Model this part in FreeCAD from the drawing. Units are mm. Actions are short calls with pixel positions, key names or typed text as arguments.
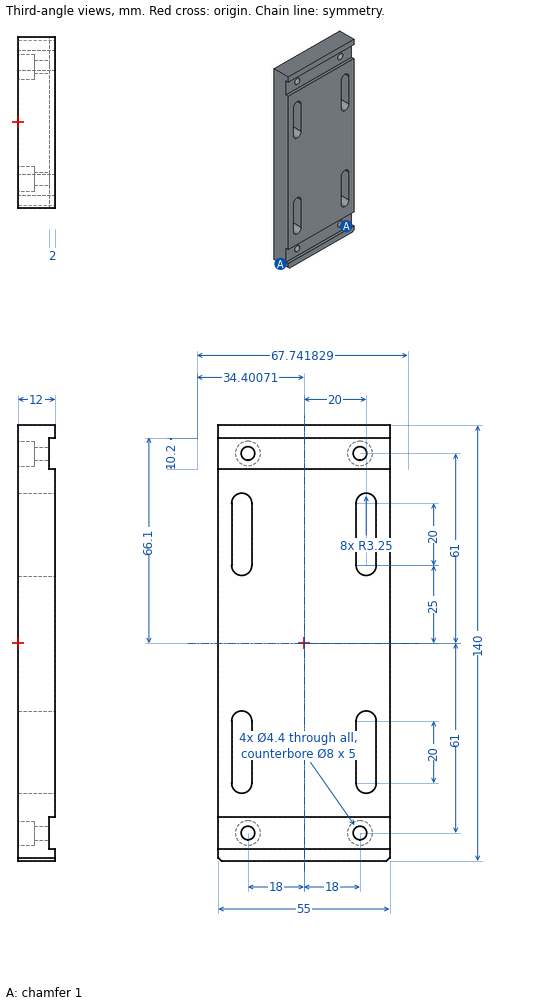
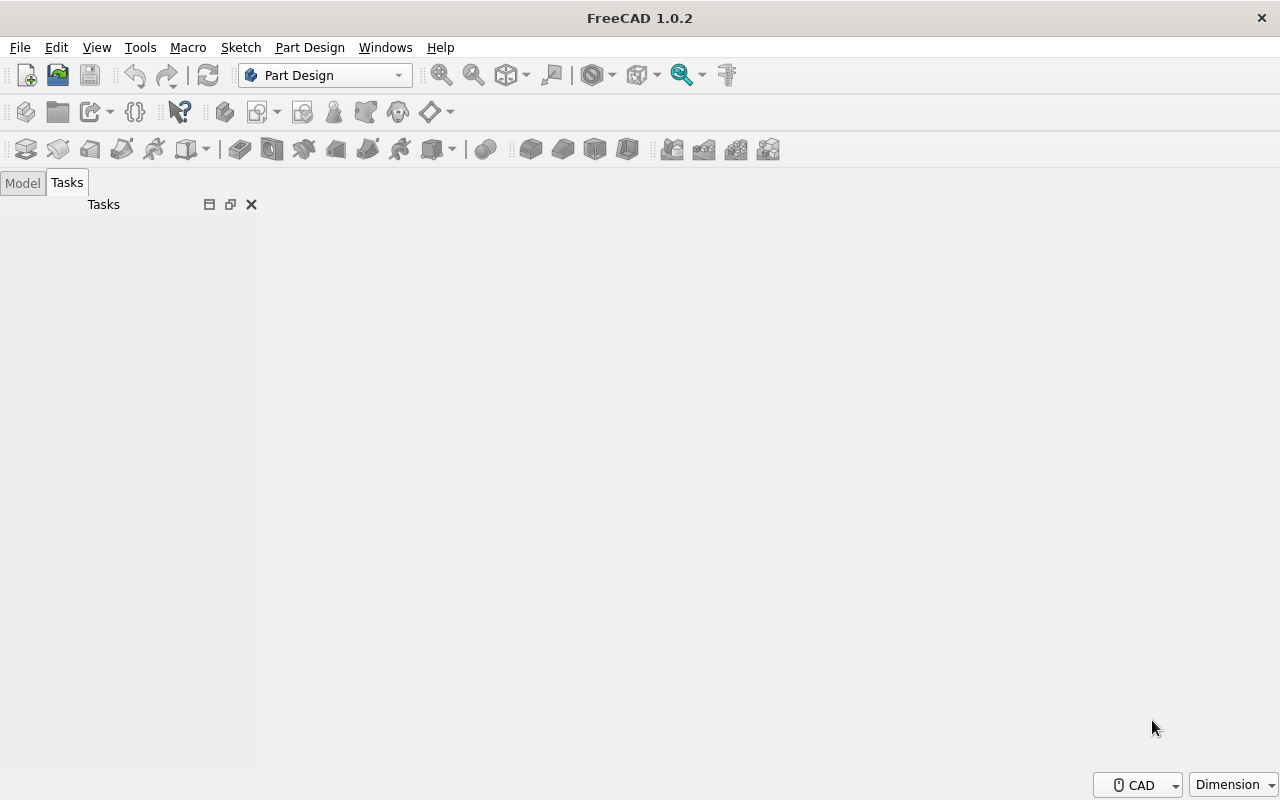
click(26, 76)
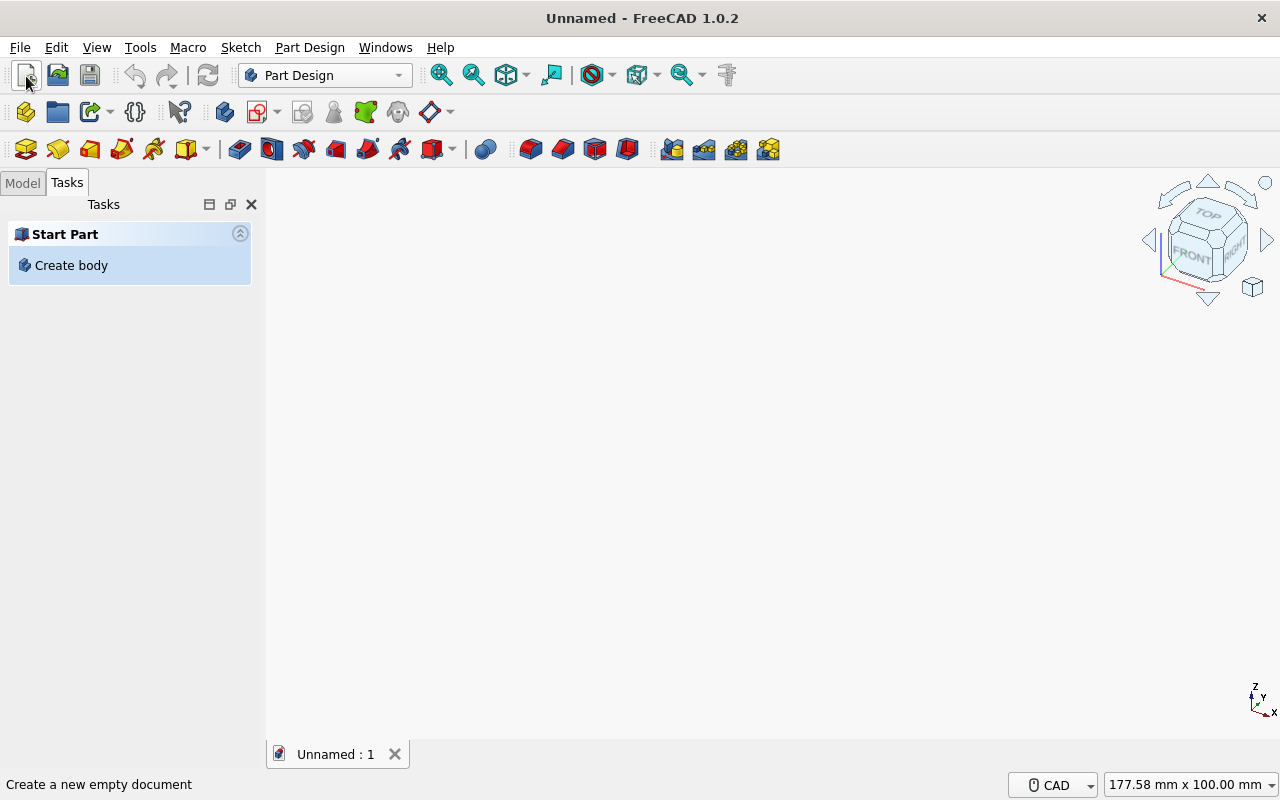
click(258, 112)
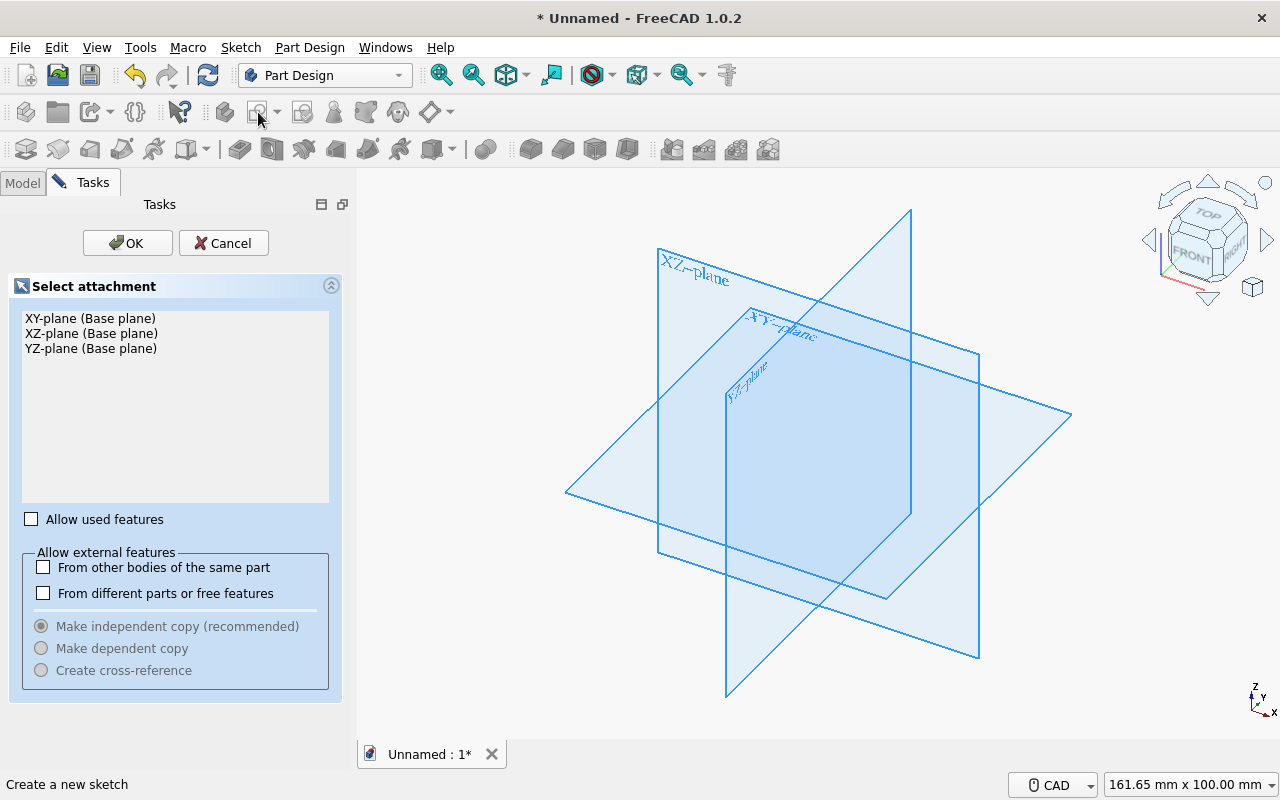
click(82, 348)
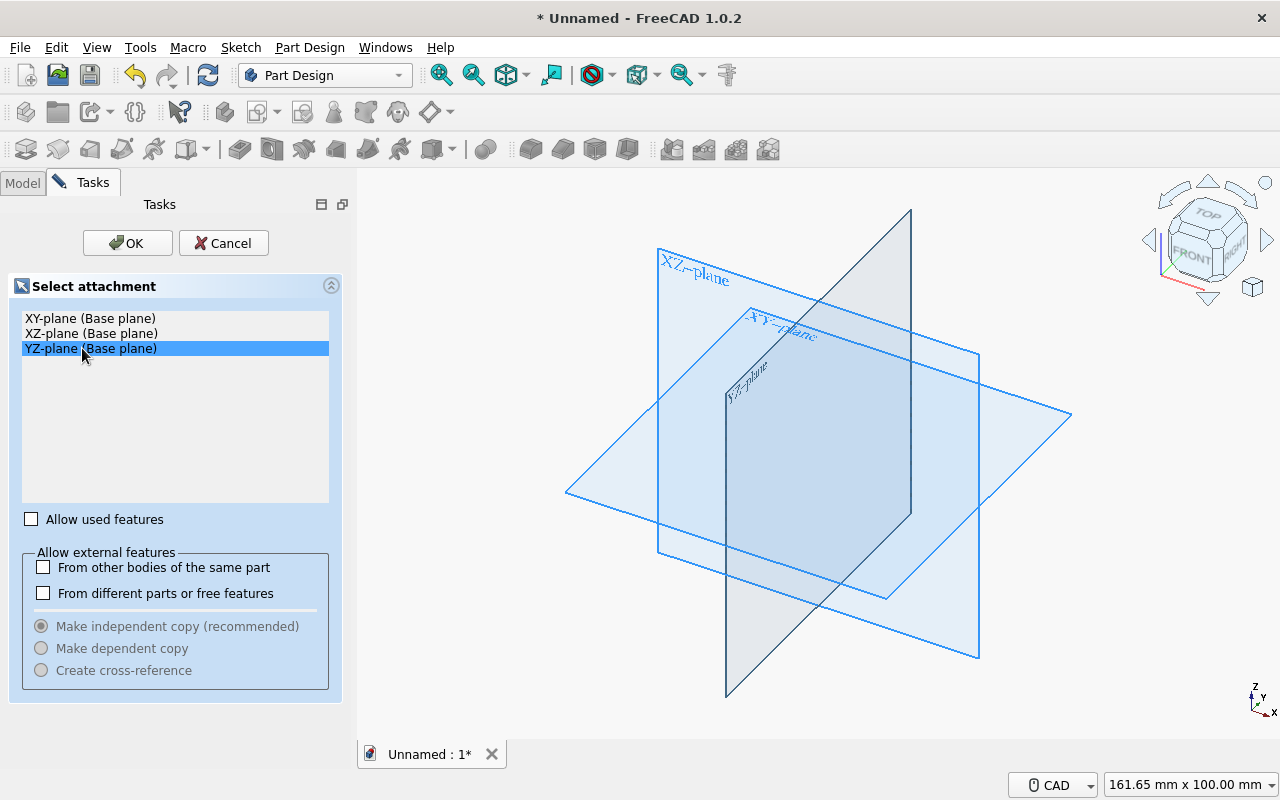
click(128, 243)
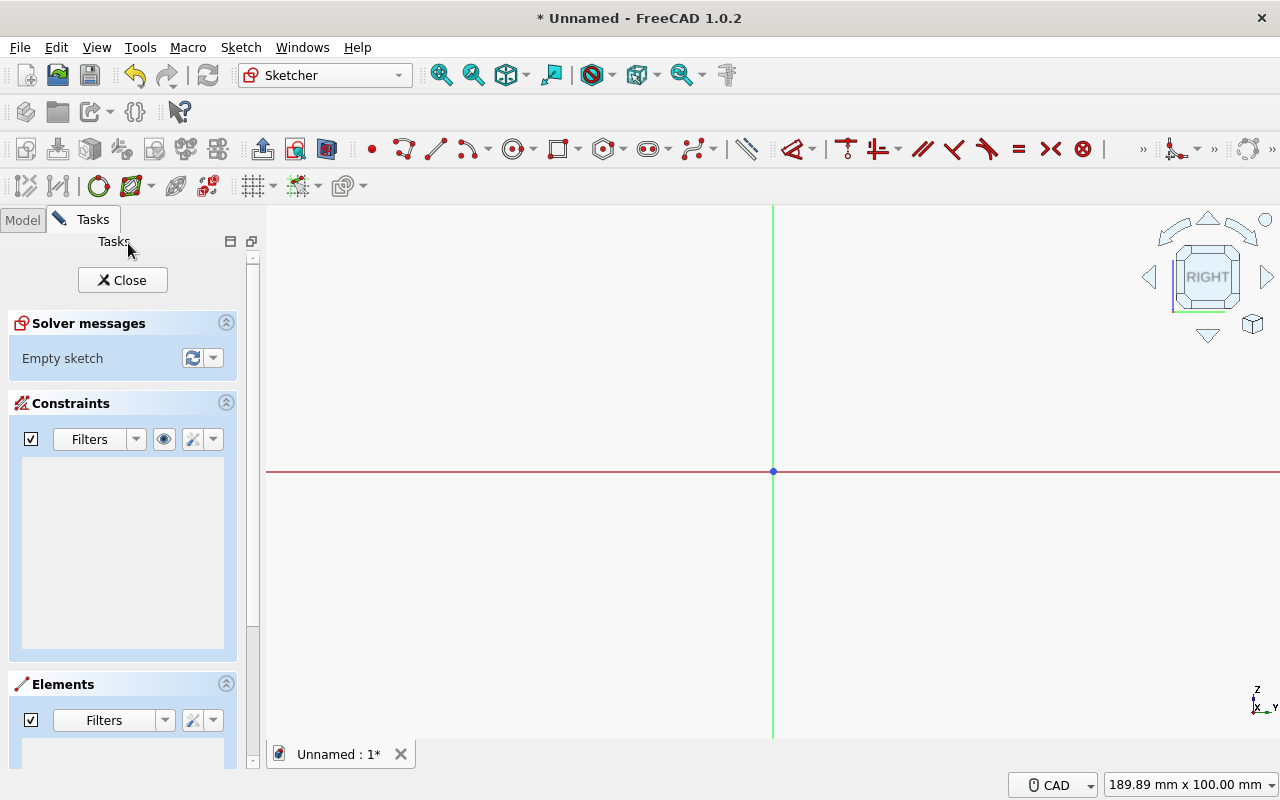
scroll(649, 472, down, 4)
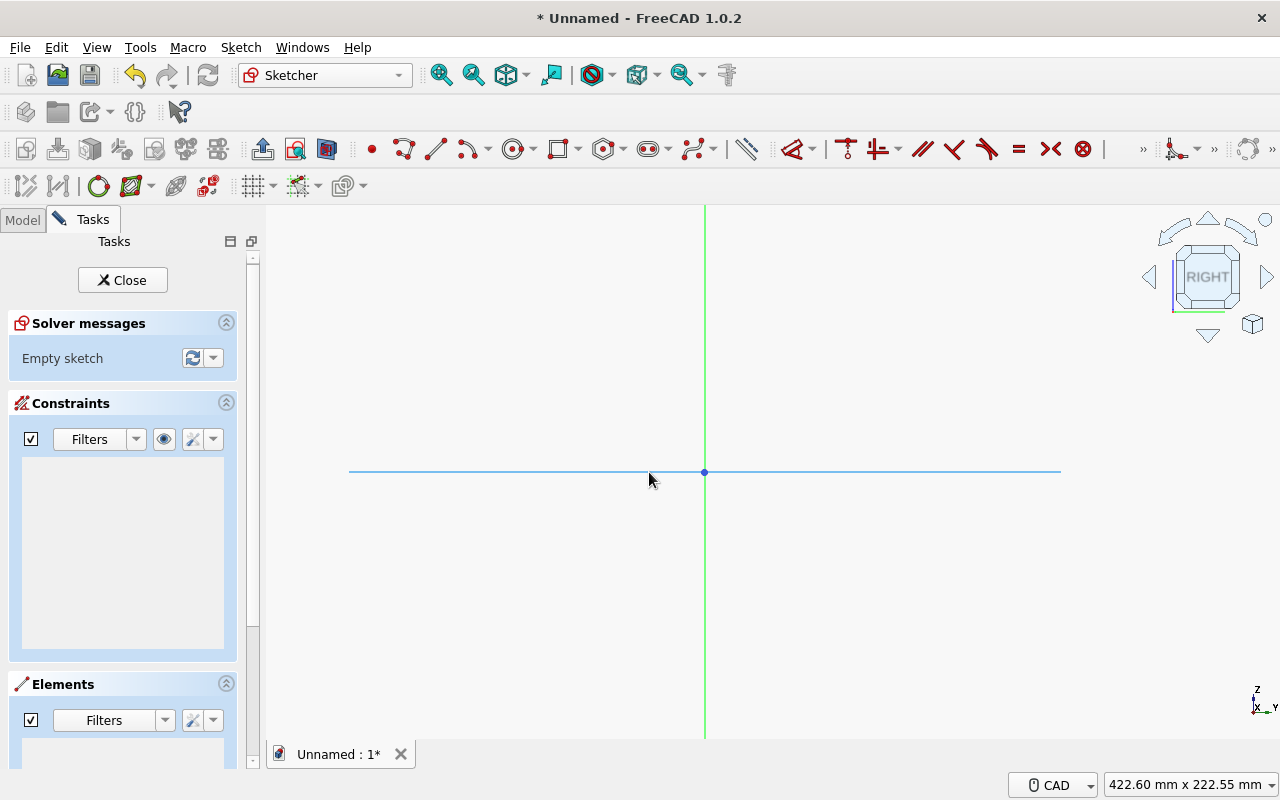
click(580, 150)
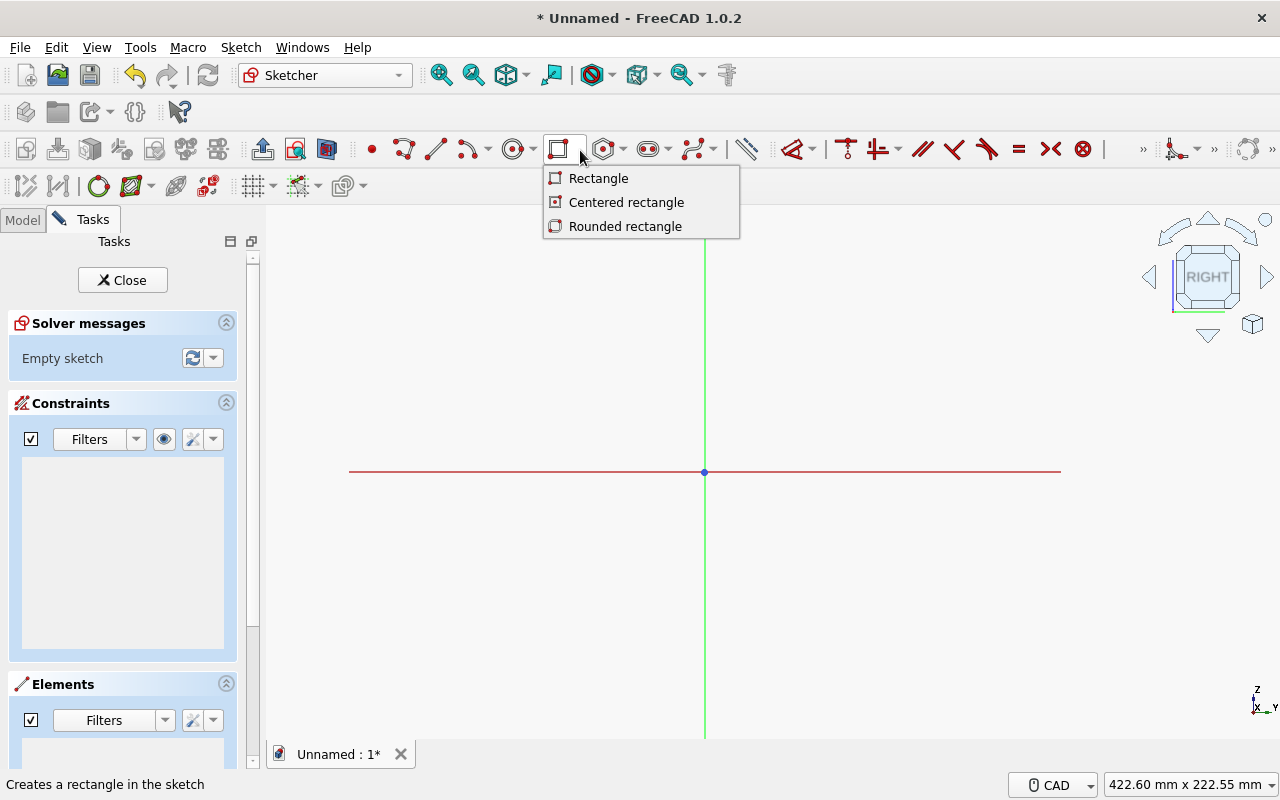
click(642, 202)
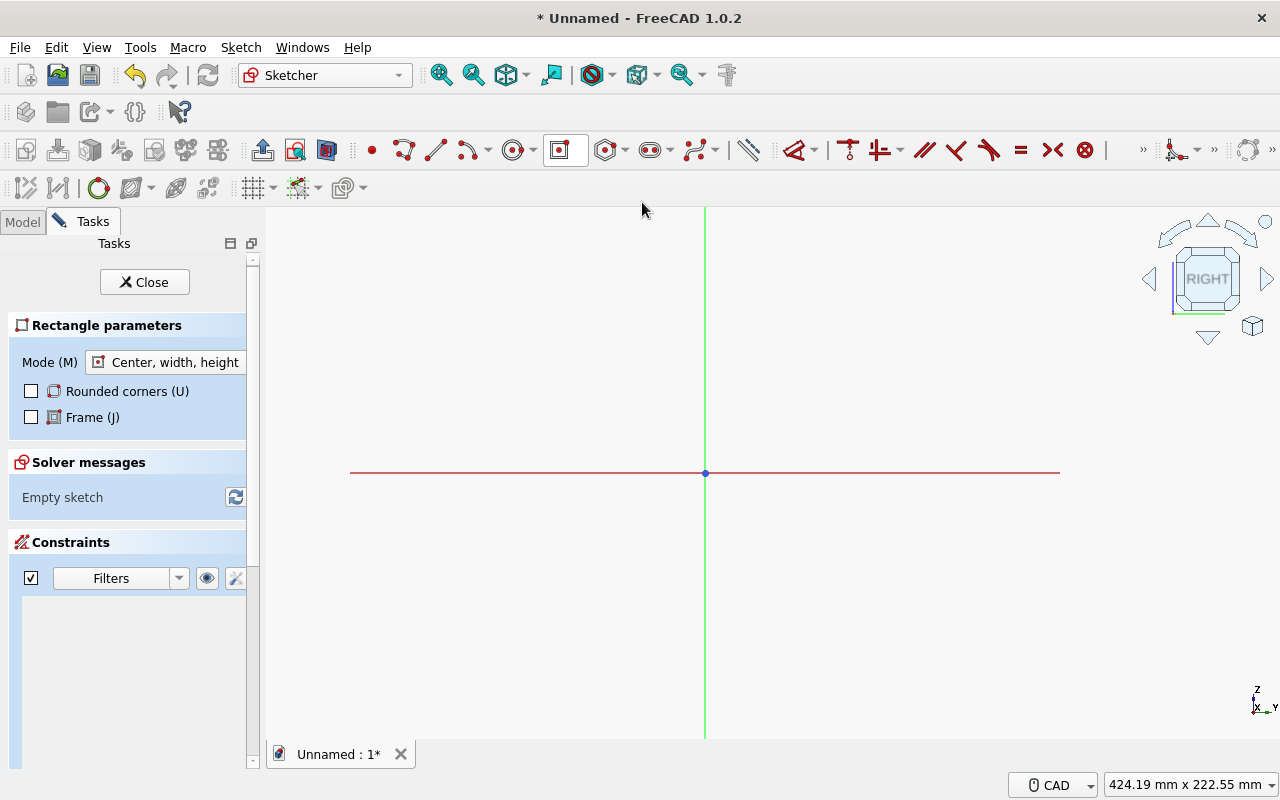
click(705, 473)
click(771, 306)
key(Escape)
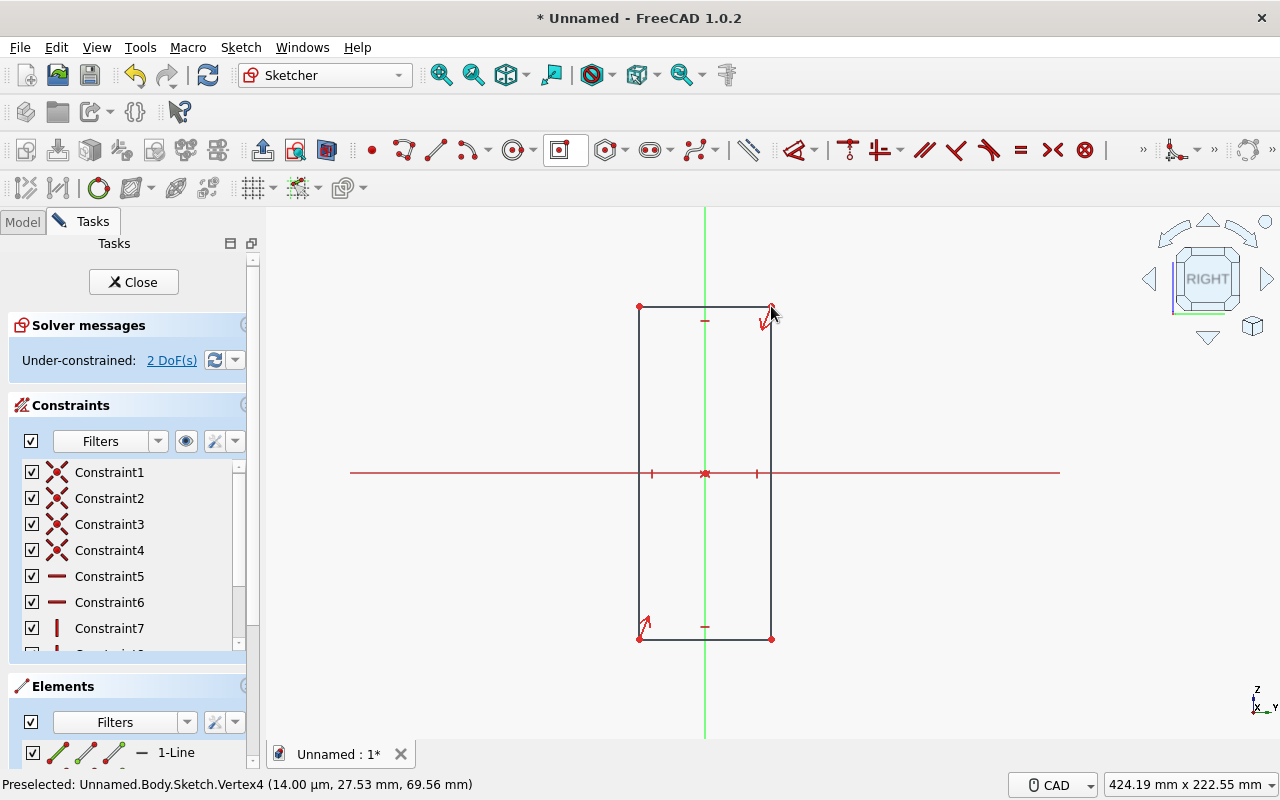
click(679, 640)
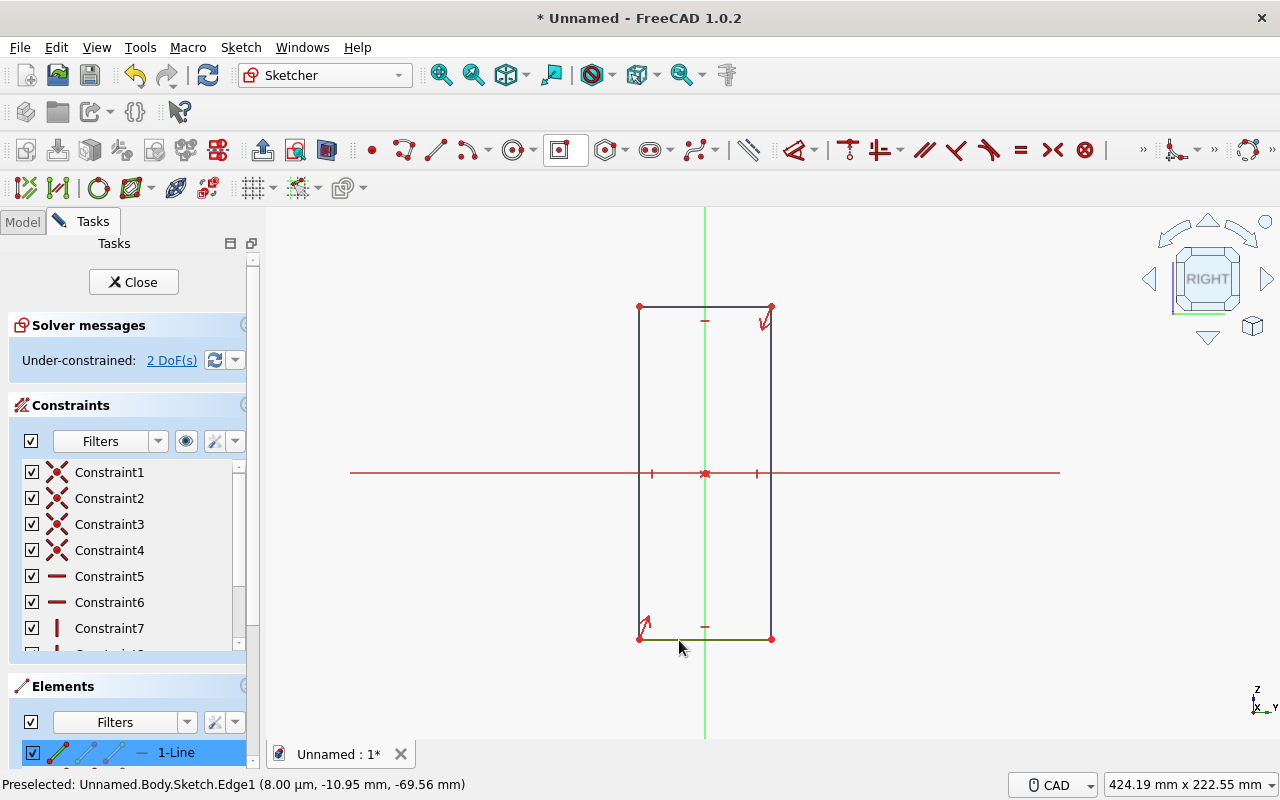
click(816, 150)